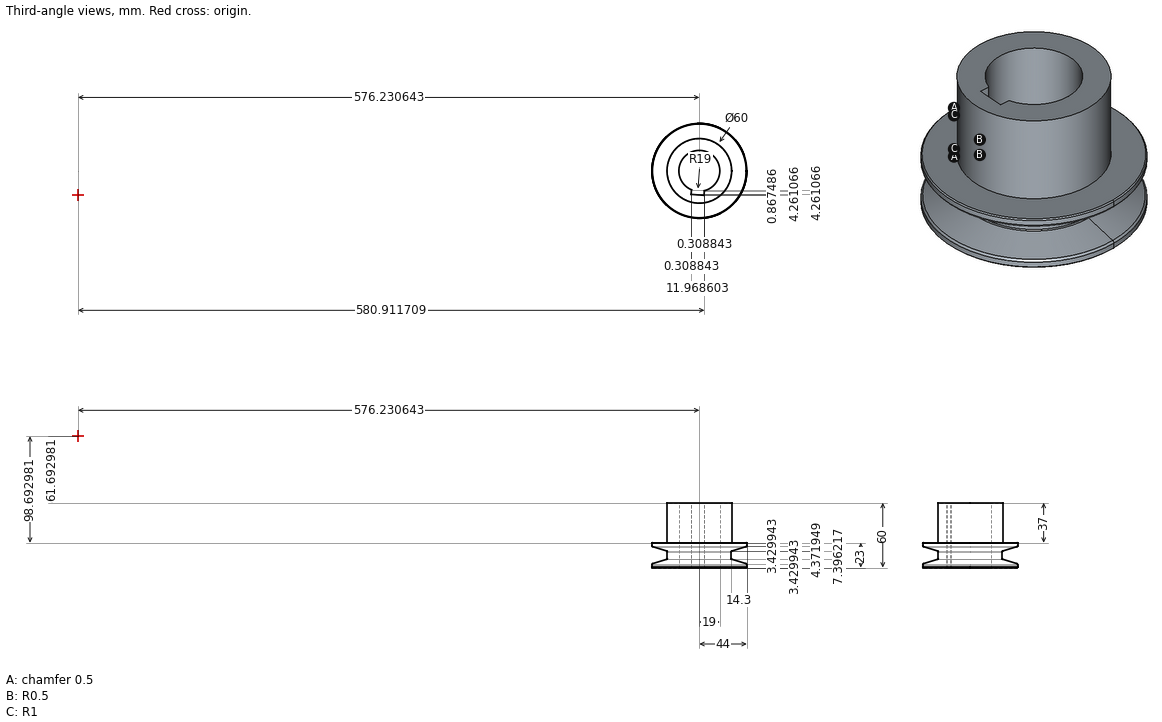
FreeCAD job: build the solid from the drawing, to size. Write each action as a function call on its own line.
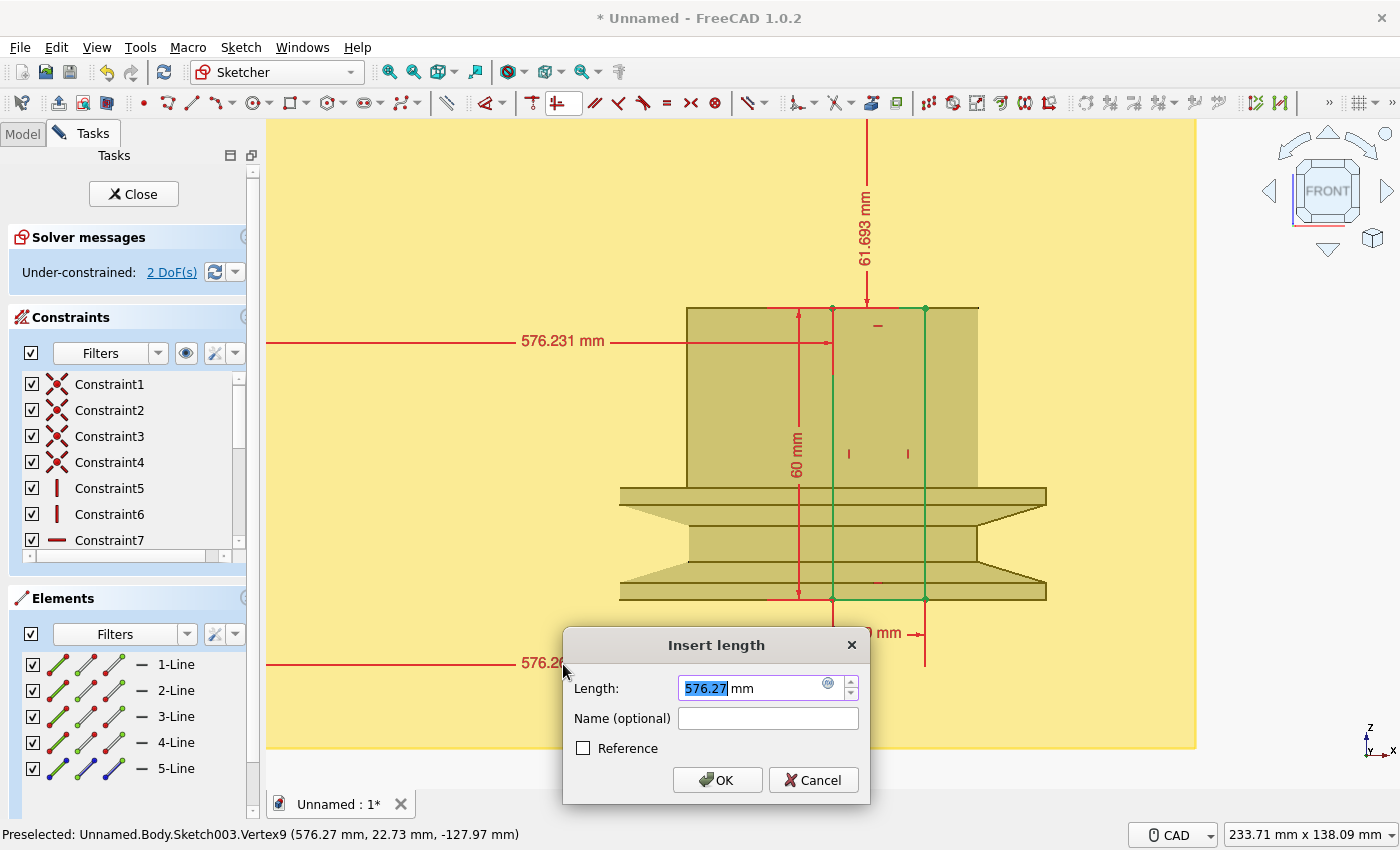
text(576.230643)
key(Return)
key(Escape)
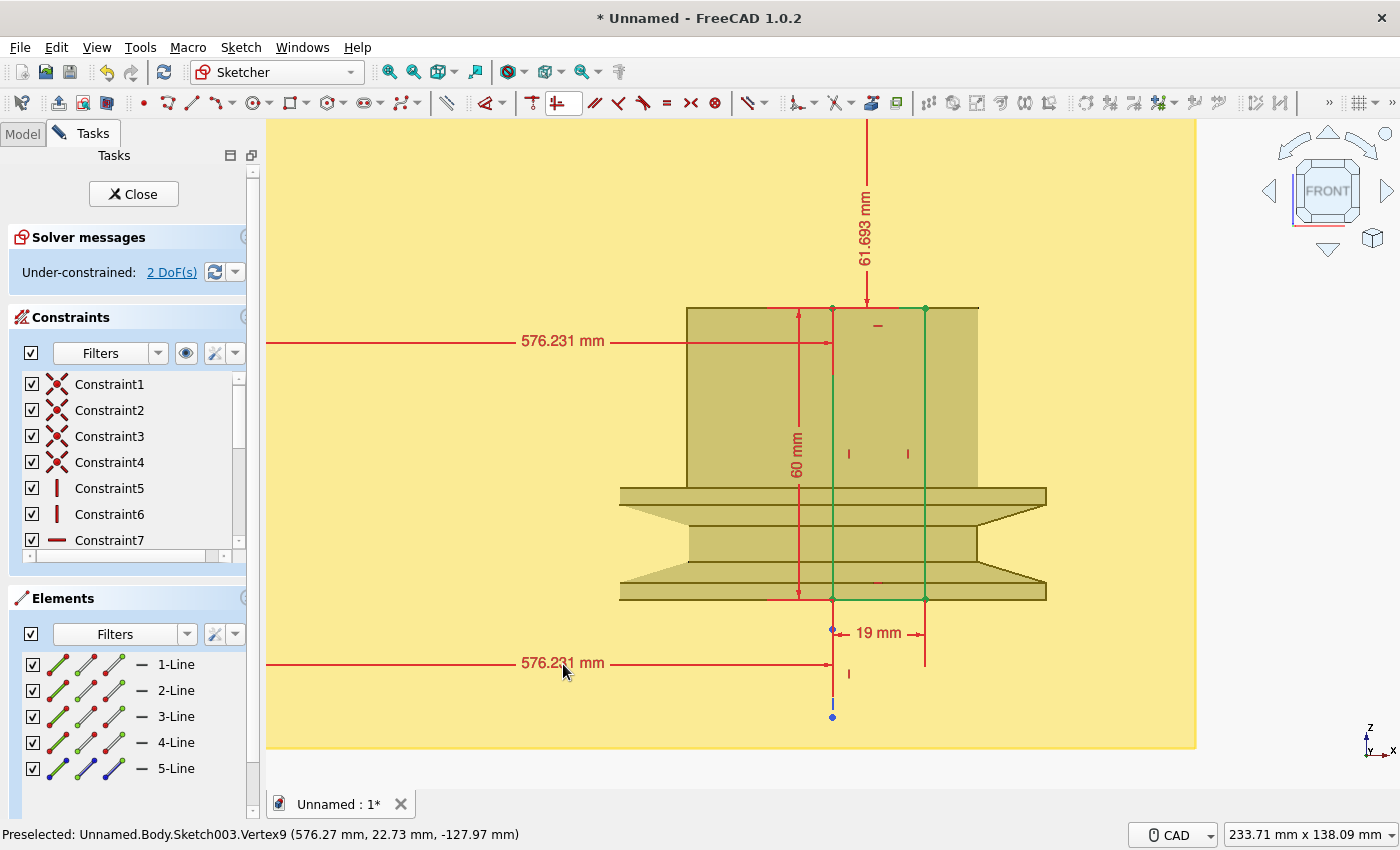
click(134, 194)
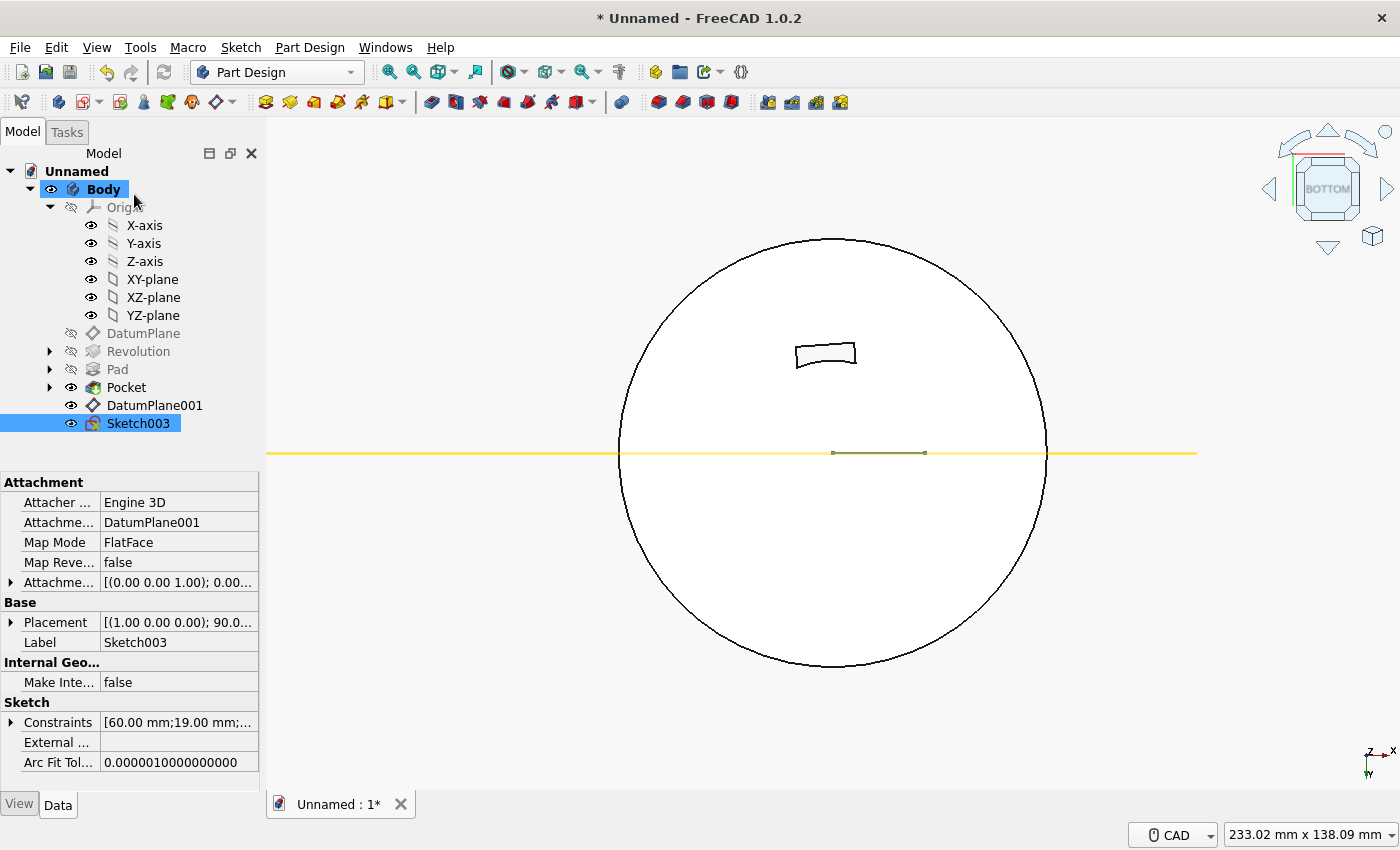
click(480, 102)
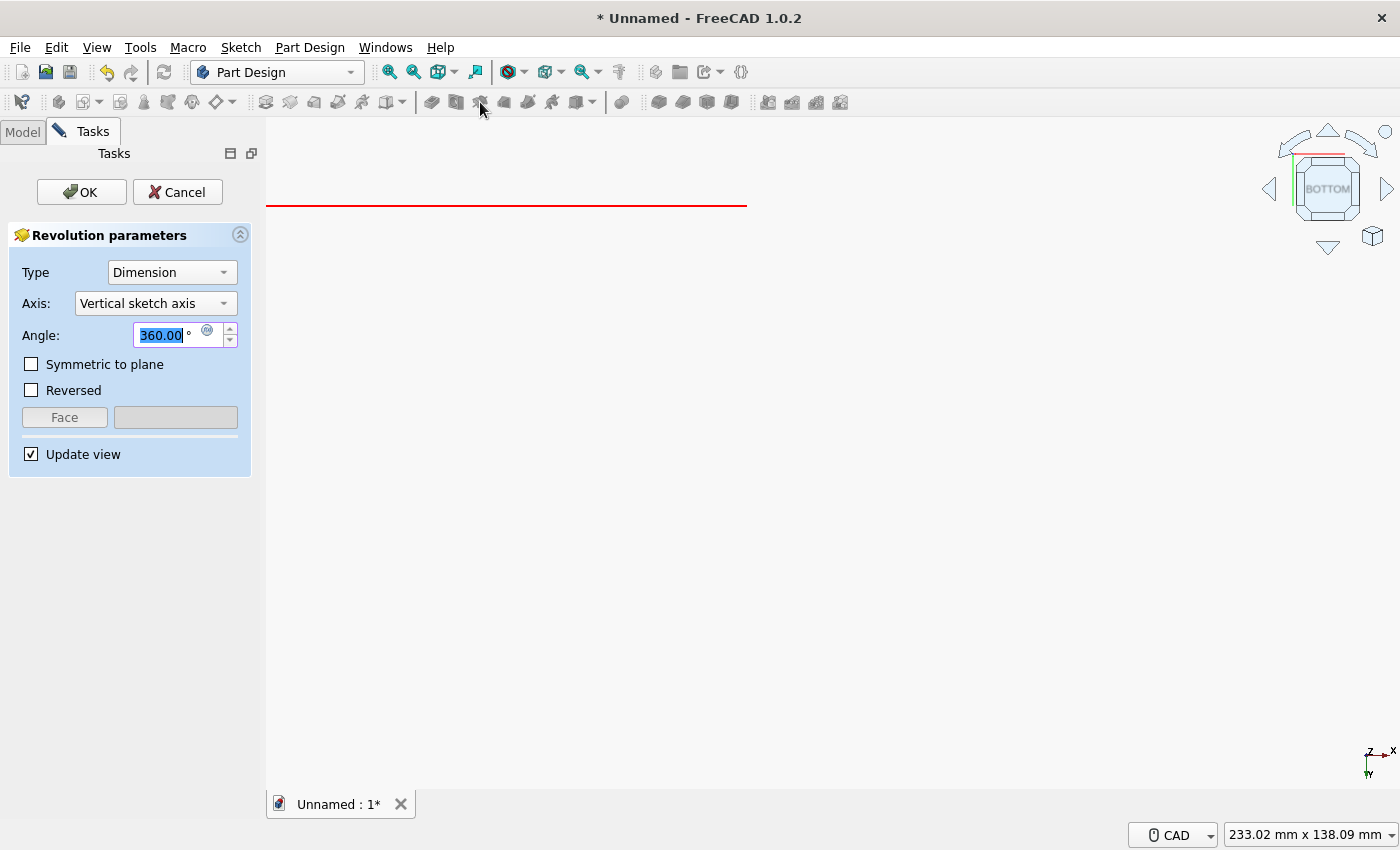
click(156, 304)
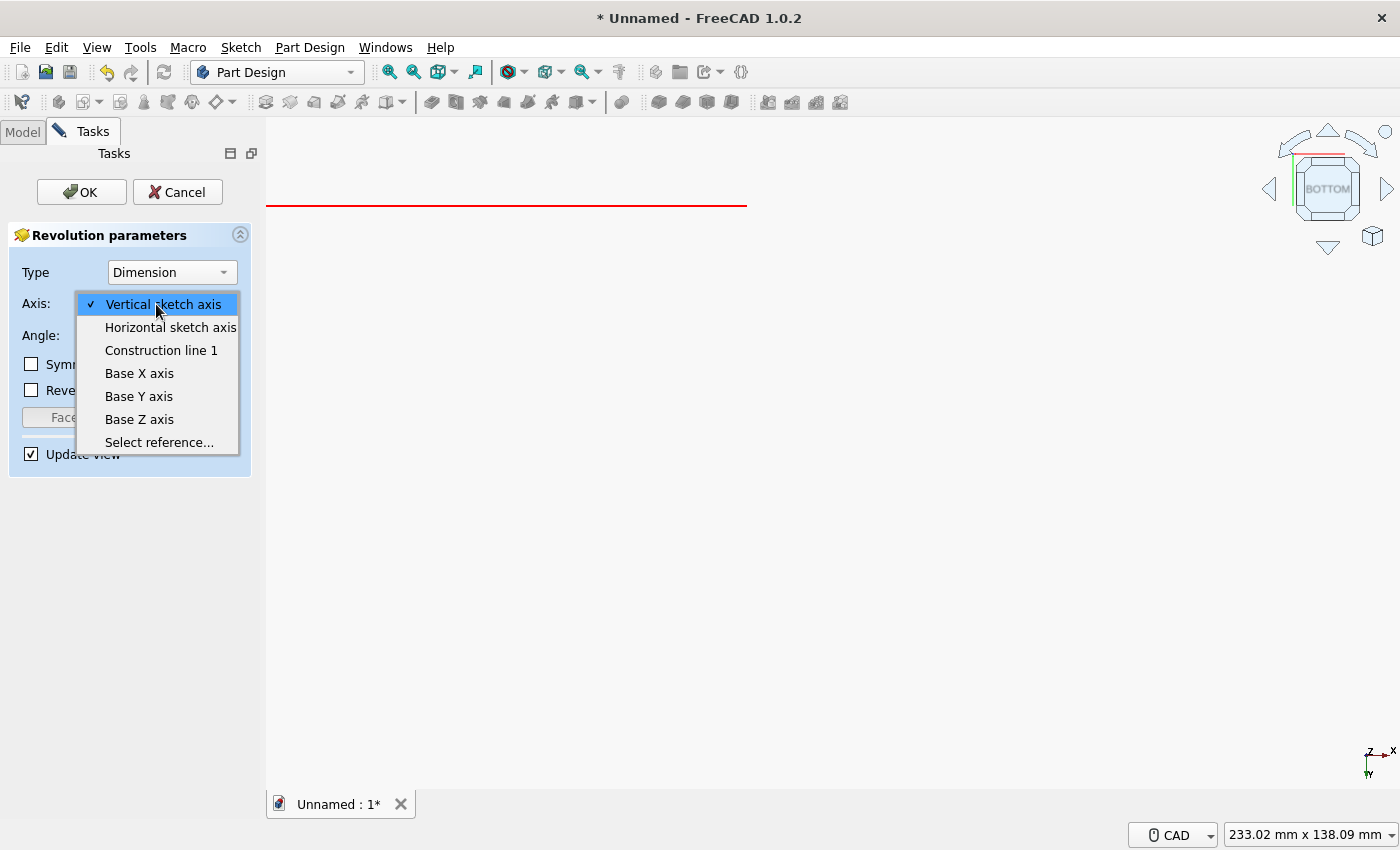
click(156, 350)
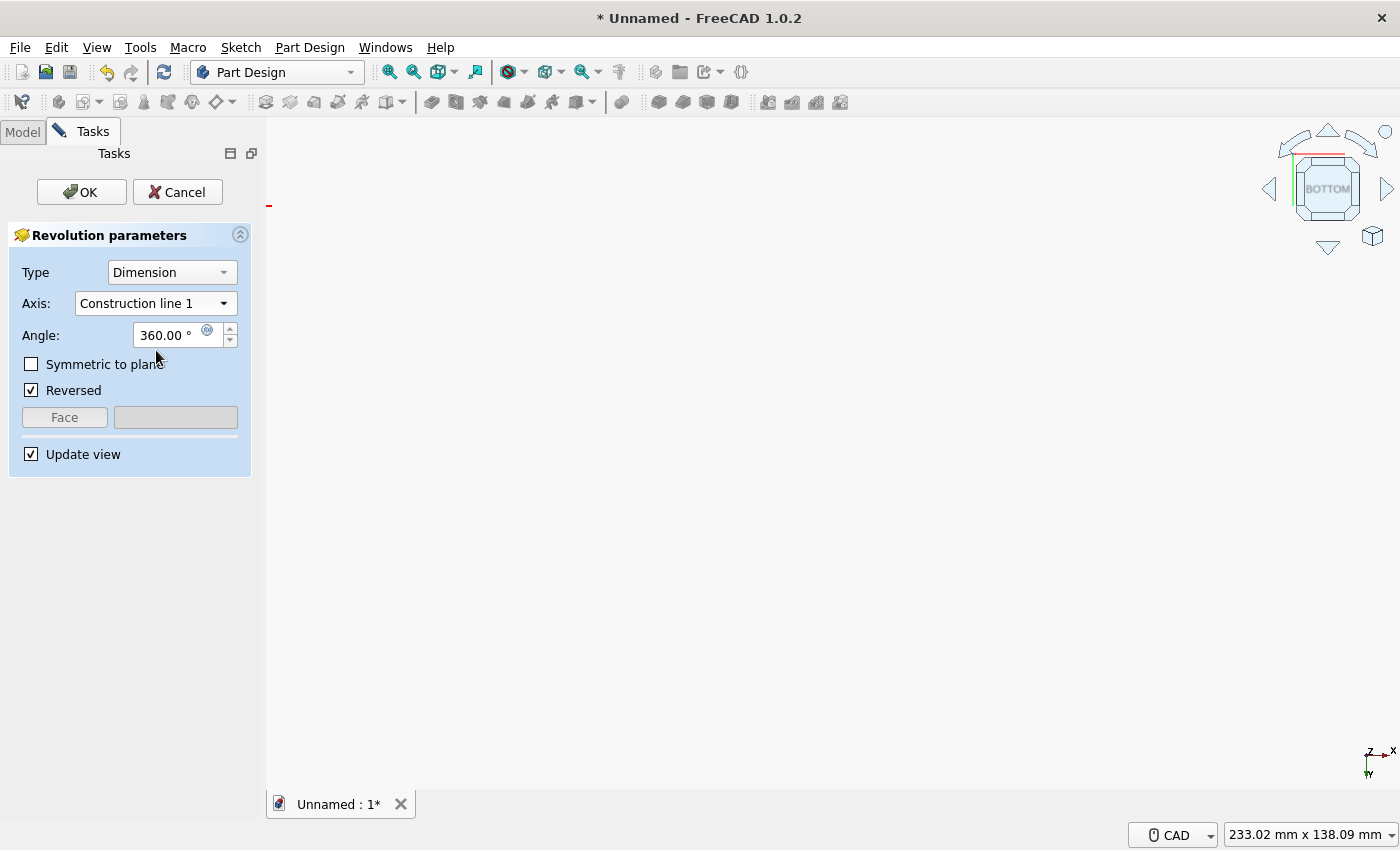
click(82, 192)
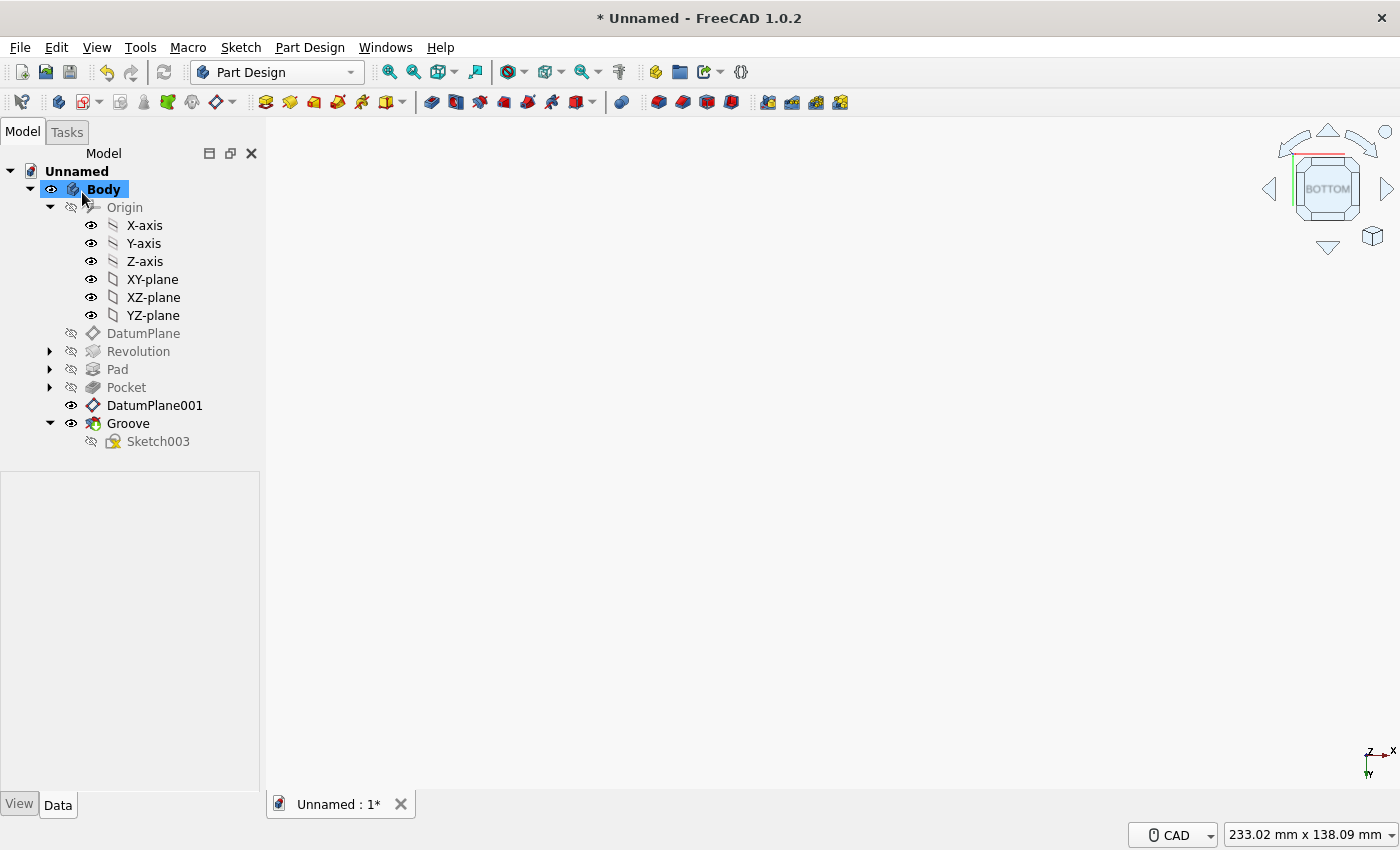
click(116, 405)
key(space)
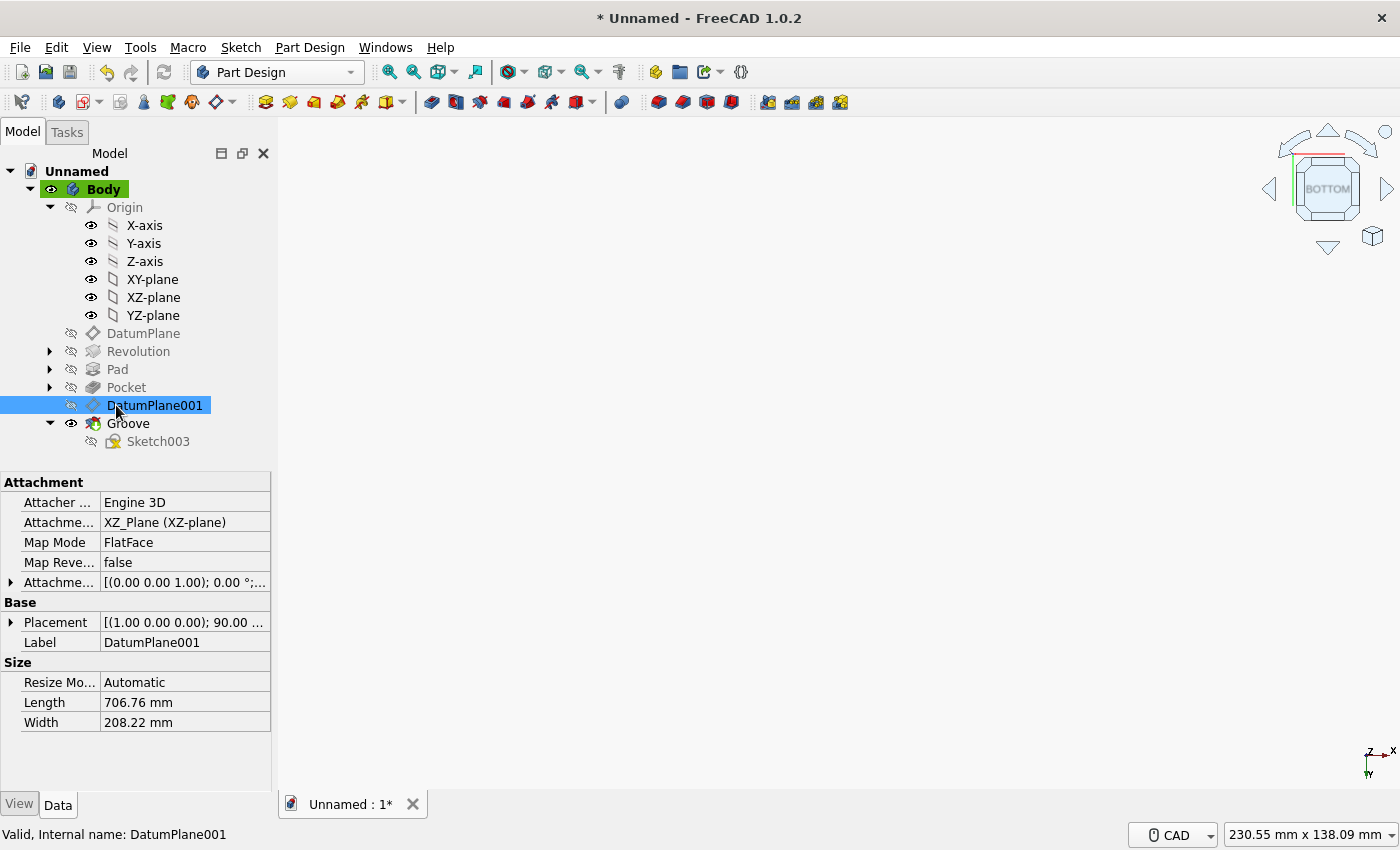
click(390, 72)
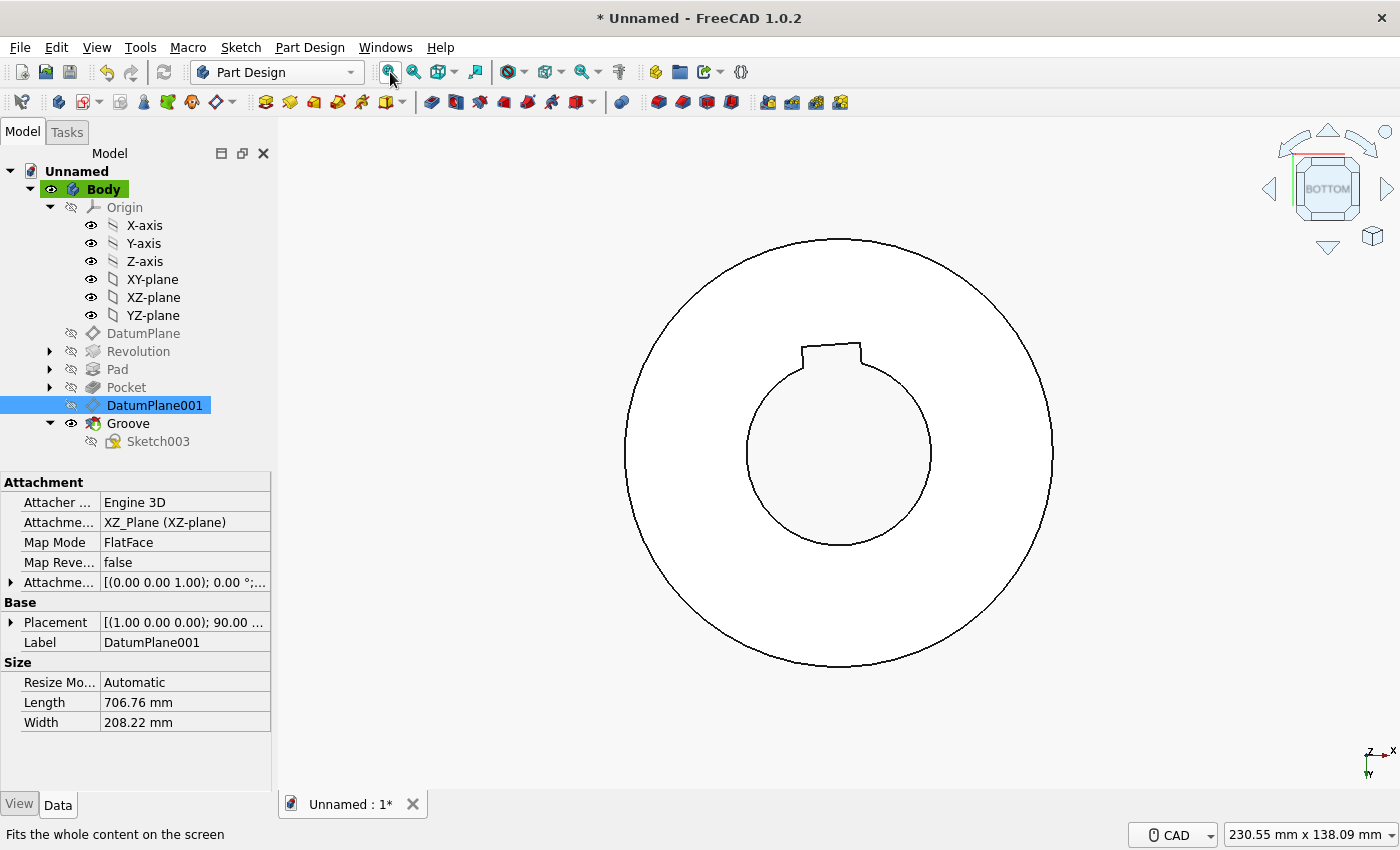
click(625, 452)